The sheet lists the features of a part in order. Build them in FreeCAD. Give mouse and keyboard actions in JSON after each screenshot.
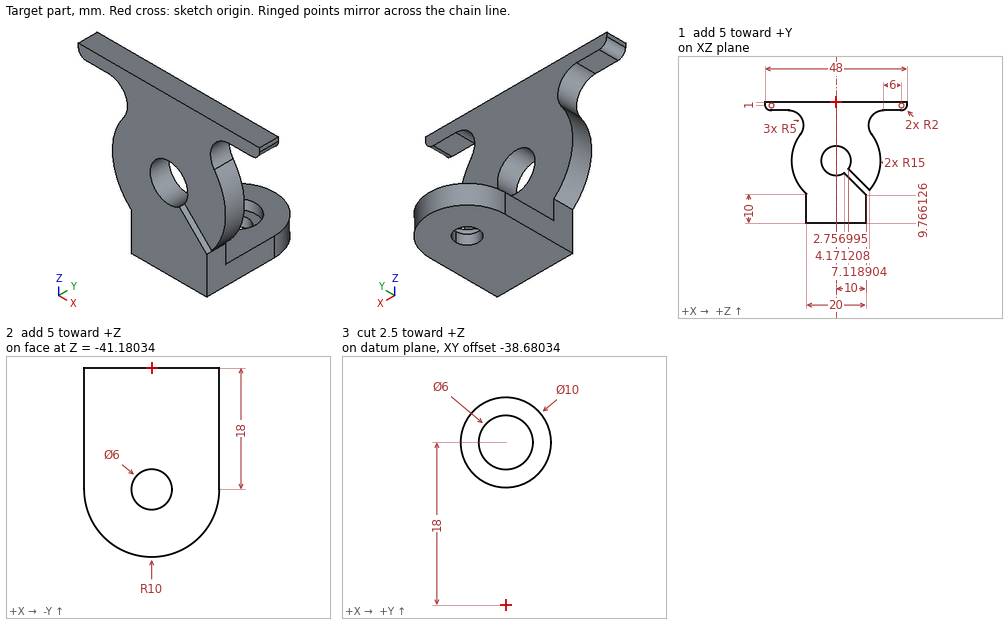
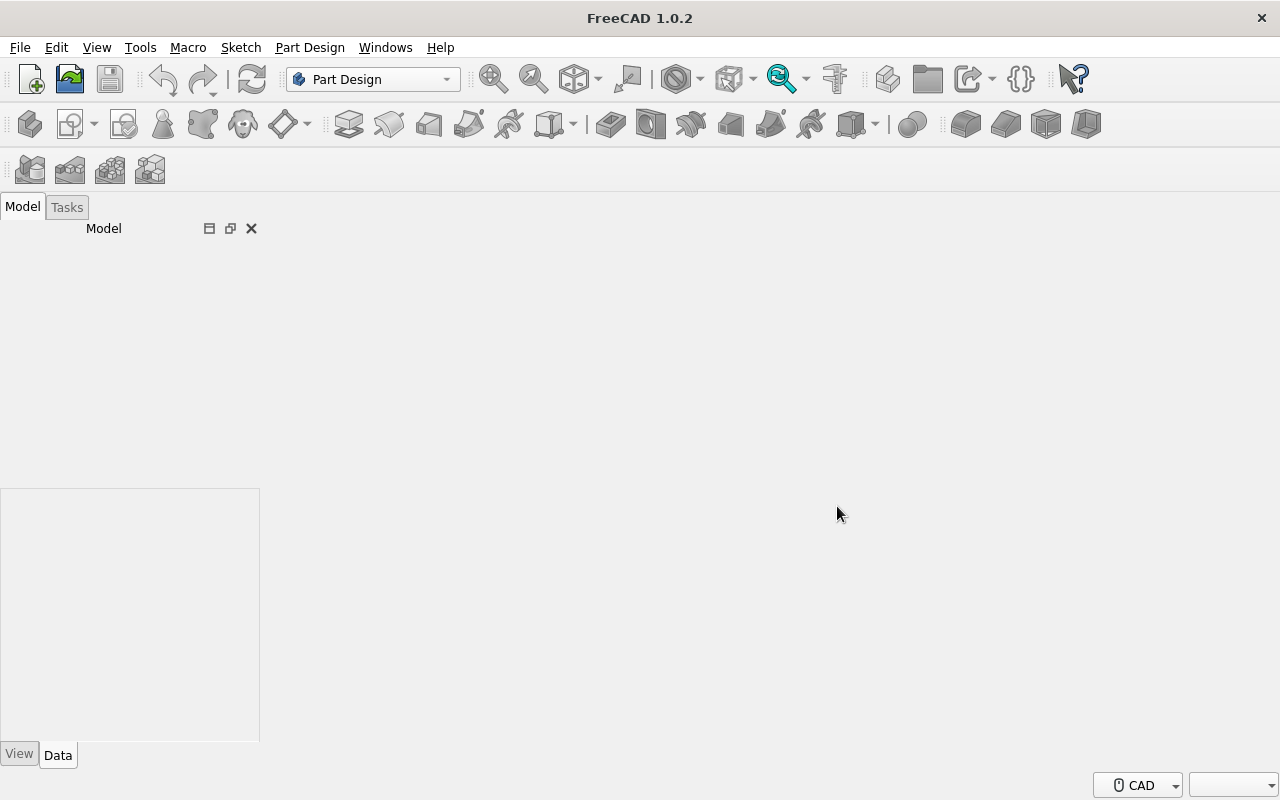
{"action": "key", "text": "ctrl+n"}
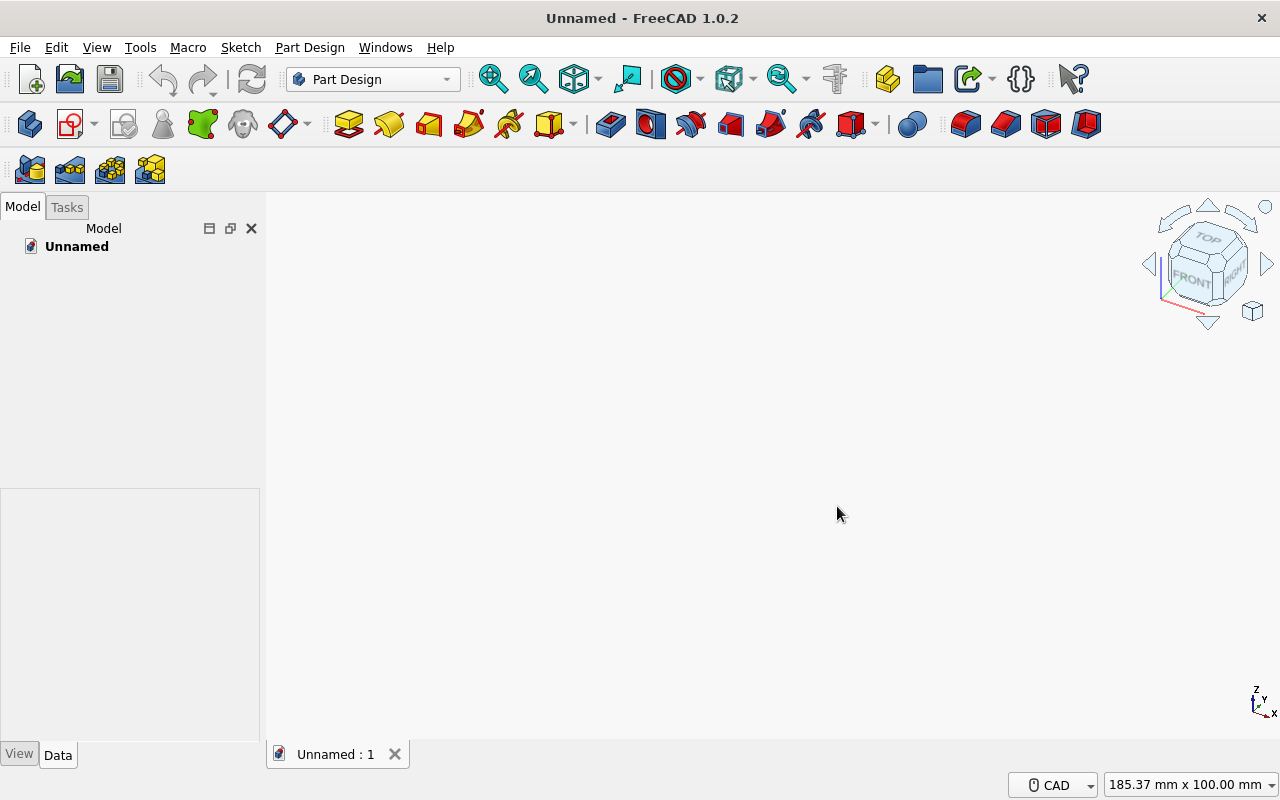
{"action": "left_click", "coordinate": [70, 124]}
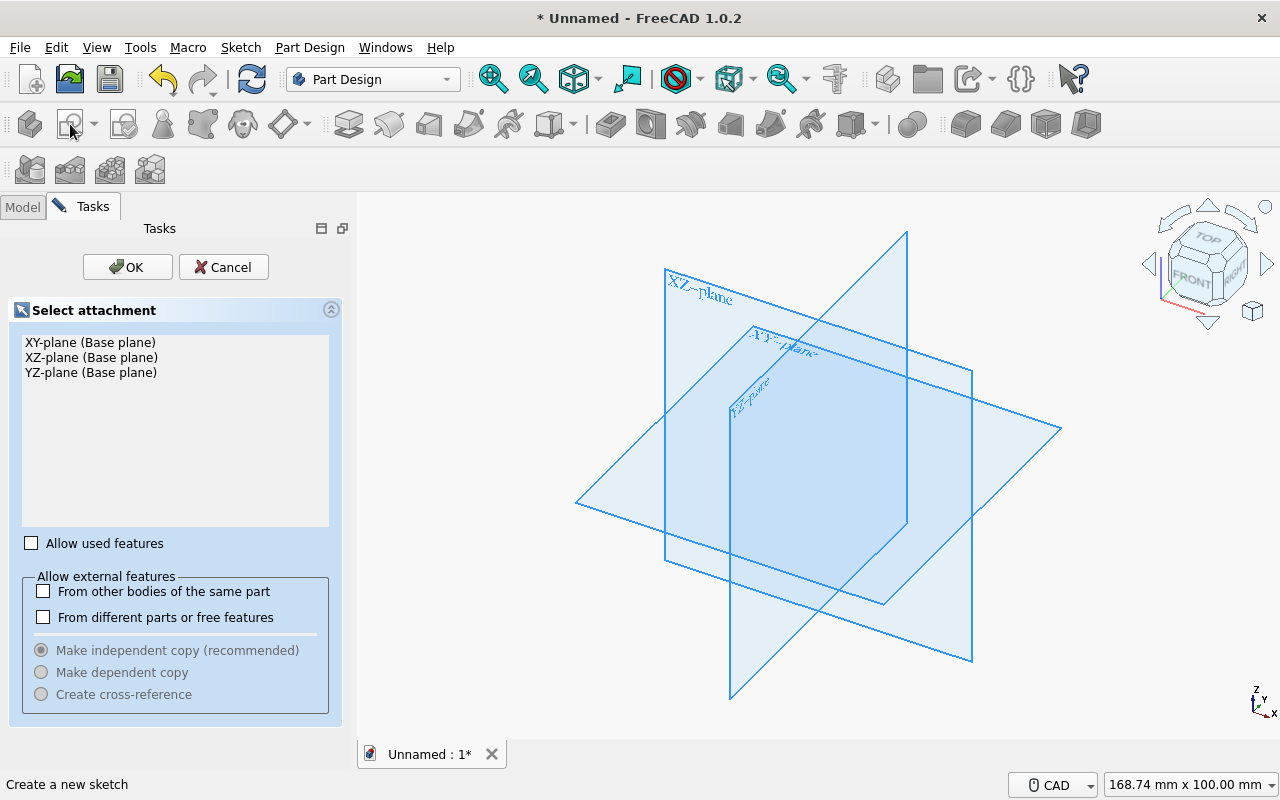
{"action": "left_click", "coordinate": [82, 358]}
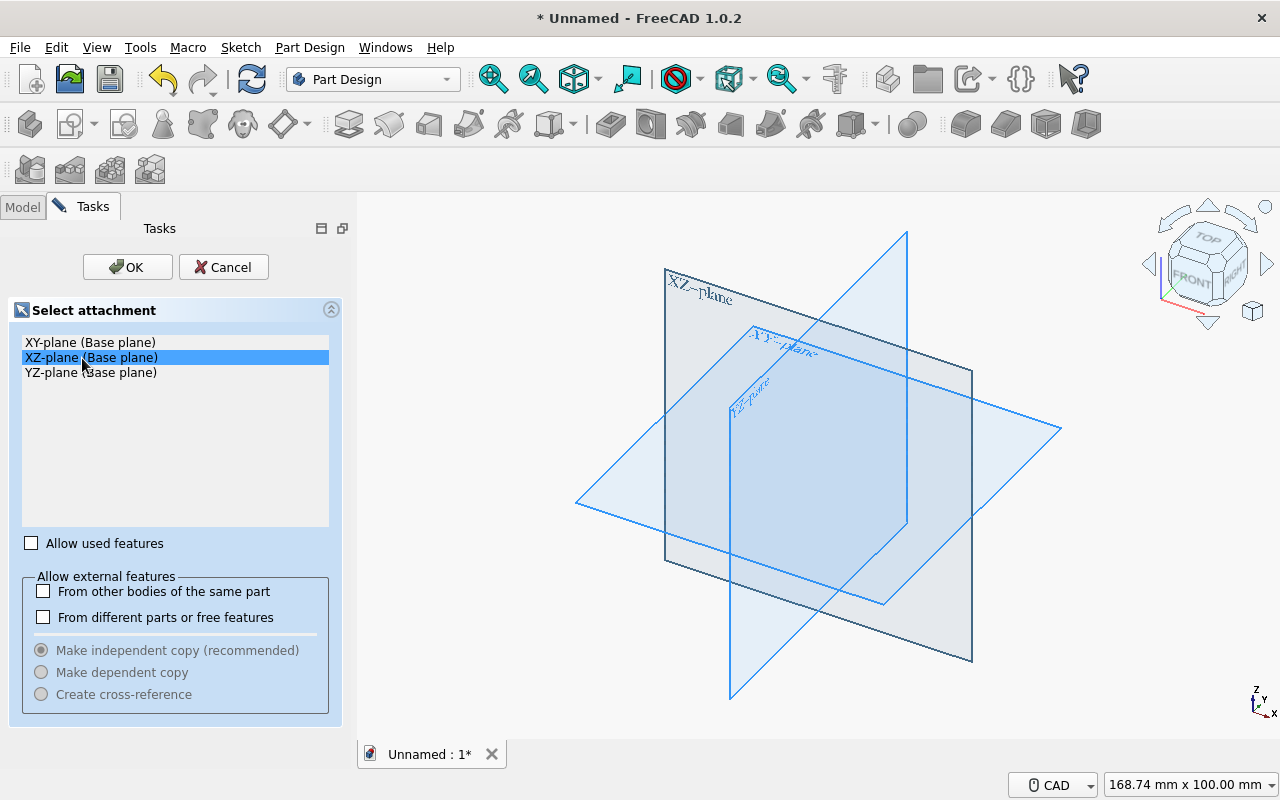
{"action": "left_click", "coordinate": [128, 267]}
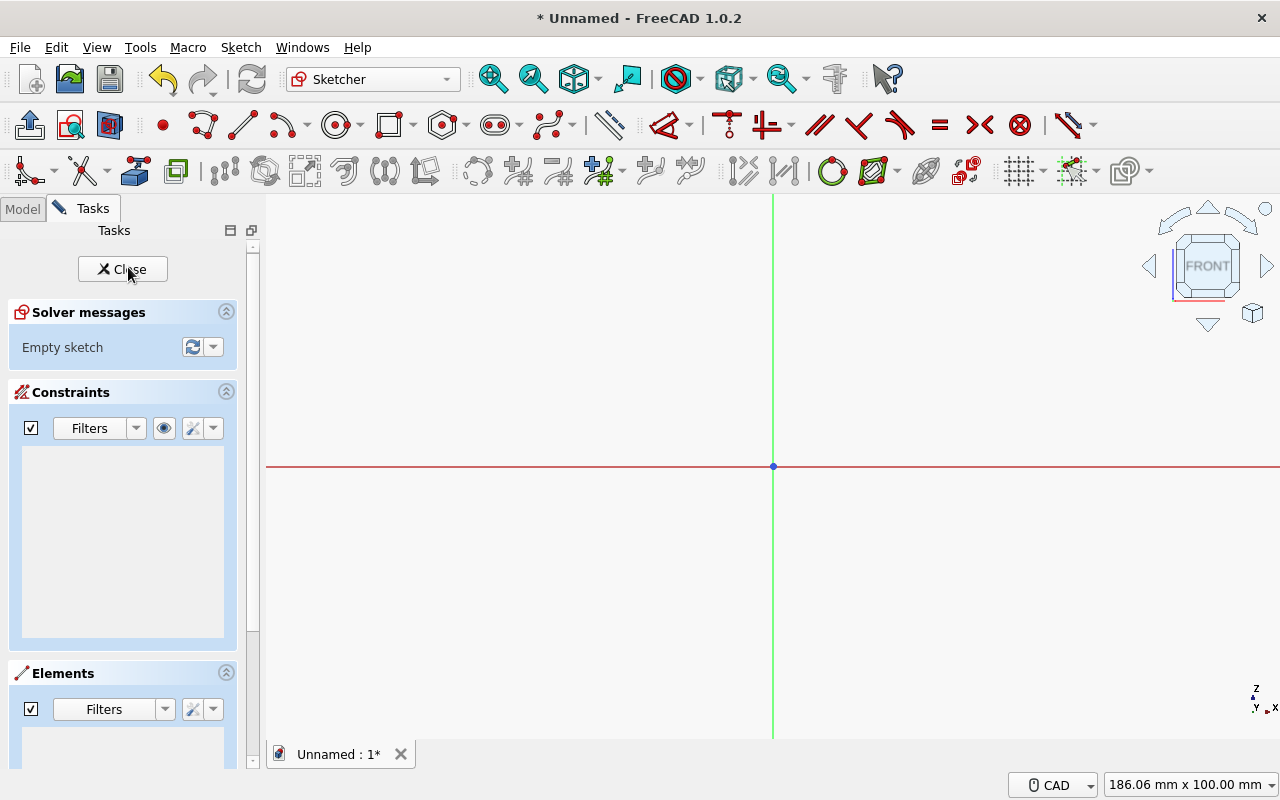
{"action": "scroll", "coordinate": [912, 711], "scroll_direction": "up", "scroll_amount": 2}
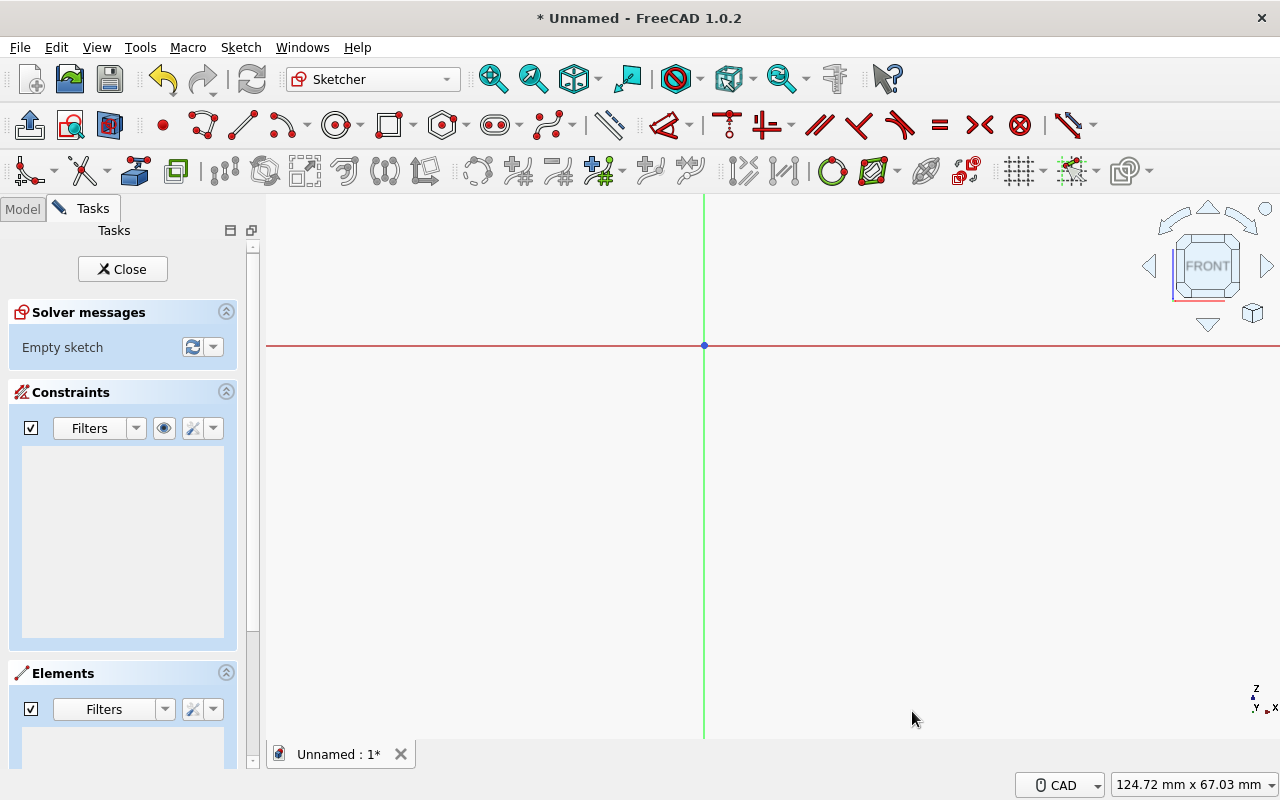
{"action": "key", "text": "g m"}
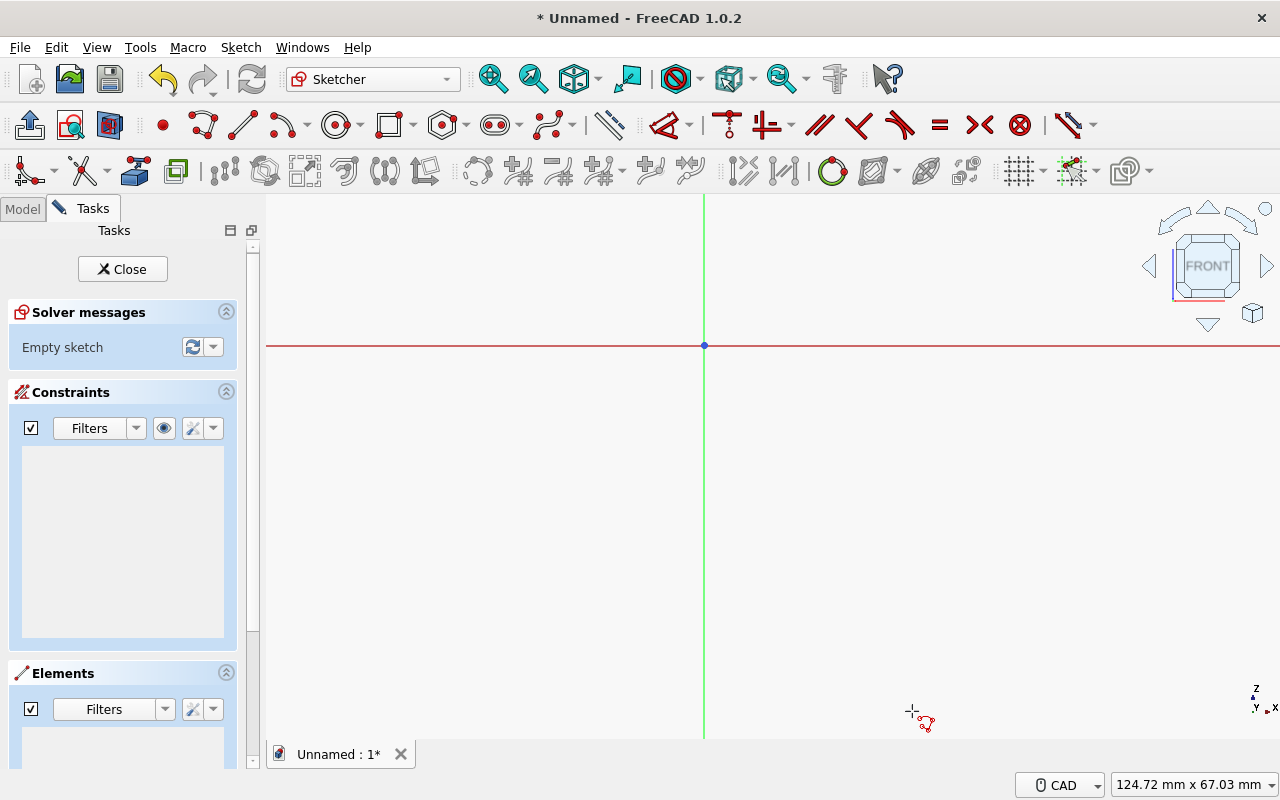
{"action": "scroll", "coordinate": [509, 354], "scroll_direction": "up", "scroll_amount": 4}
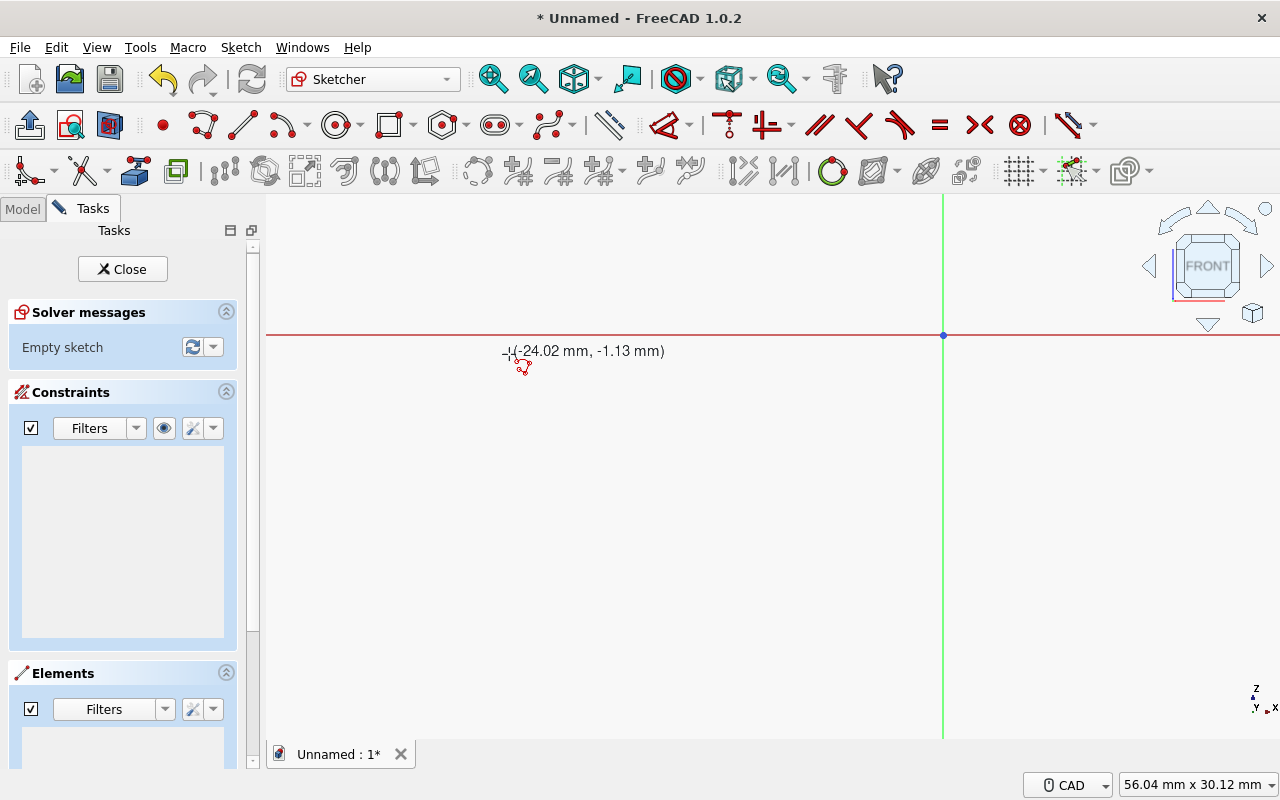
{"action": "left_click", "coordinate": [509, 353]}
{"action": "left_click", "coordinate": [509, 335]}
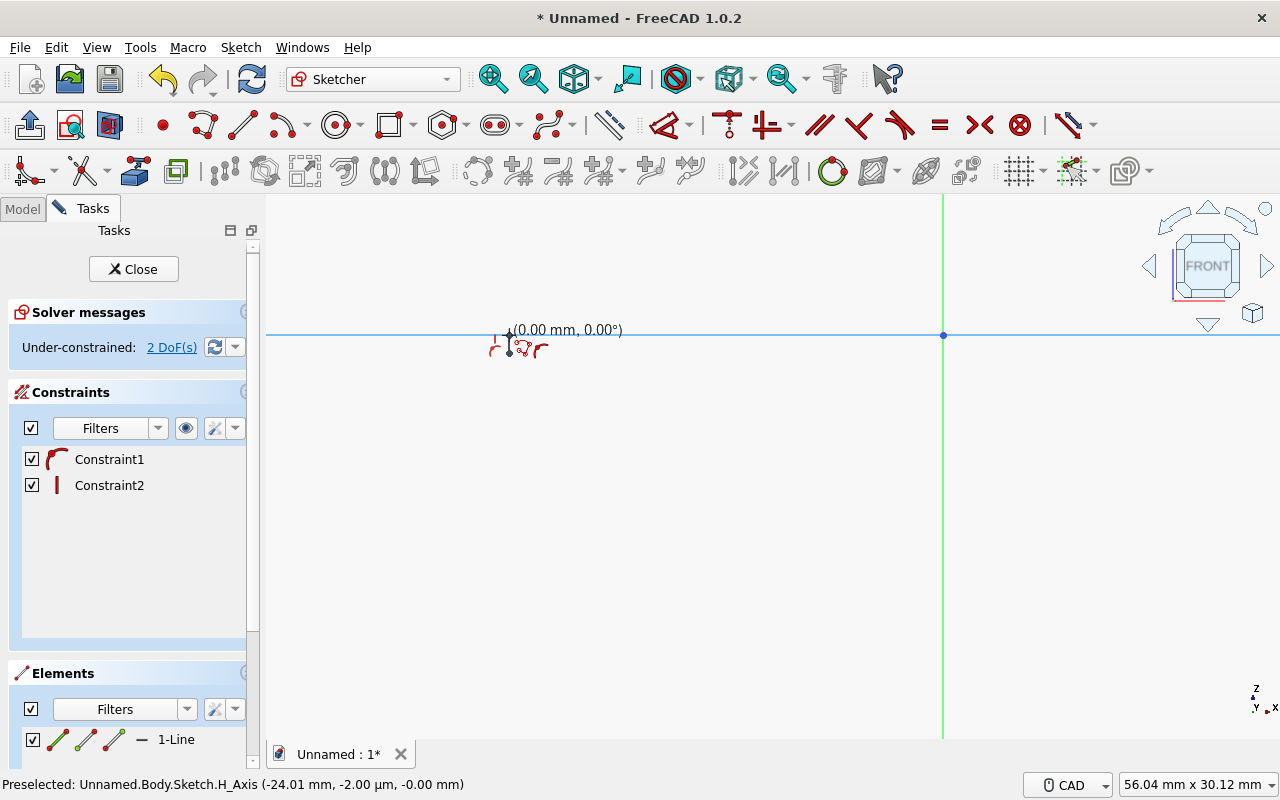
{"action": "scroll", "coordinate": [510, 270], "scroll_direction": "down", "scroll_amount": 4}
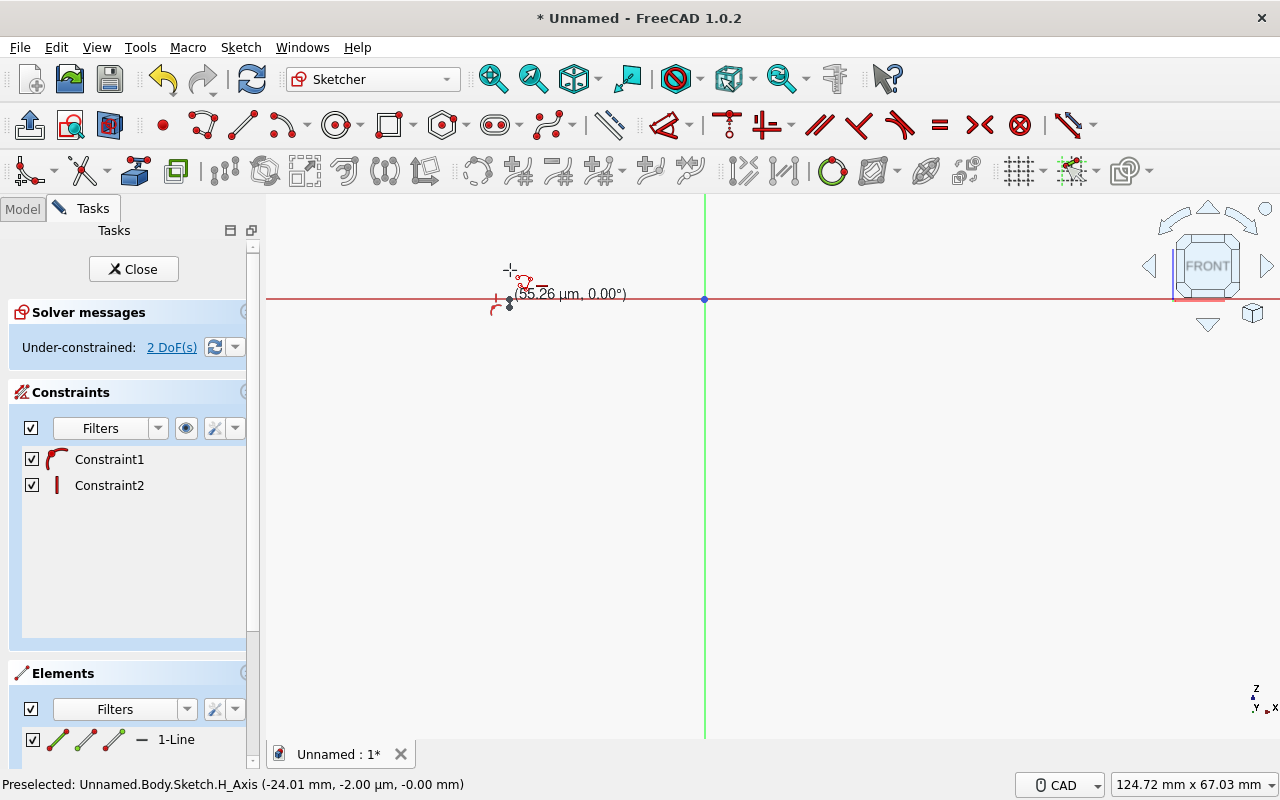
{"action": "left_click", "coordinate": [900, 308]}